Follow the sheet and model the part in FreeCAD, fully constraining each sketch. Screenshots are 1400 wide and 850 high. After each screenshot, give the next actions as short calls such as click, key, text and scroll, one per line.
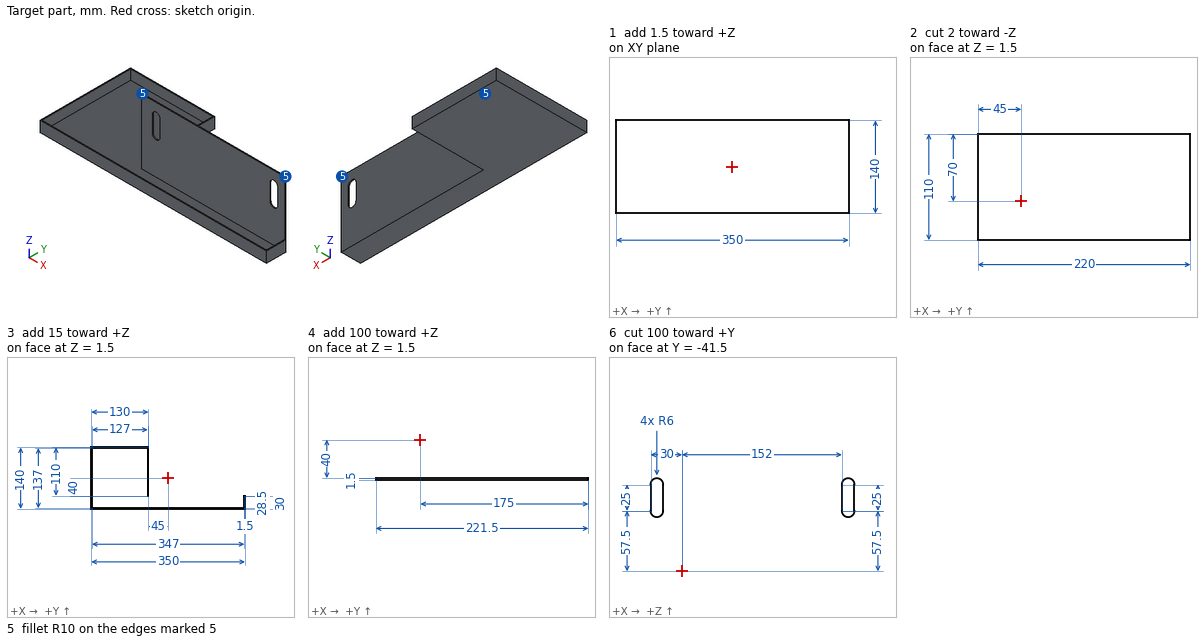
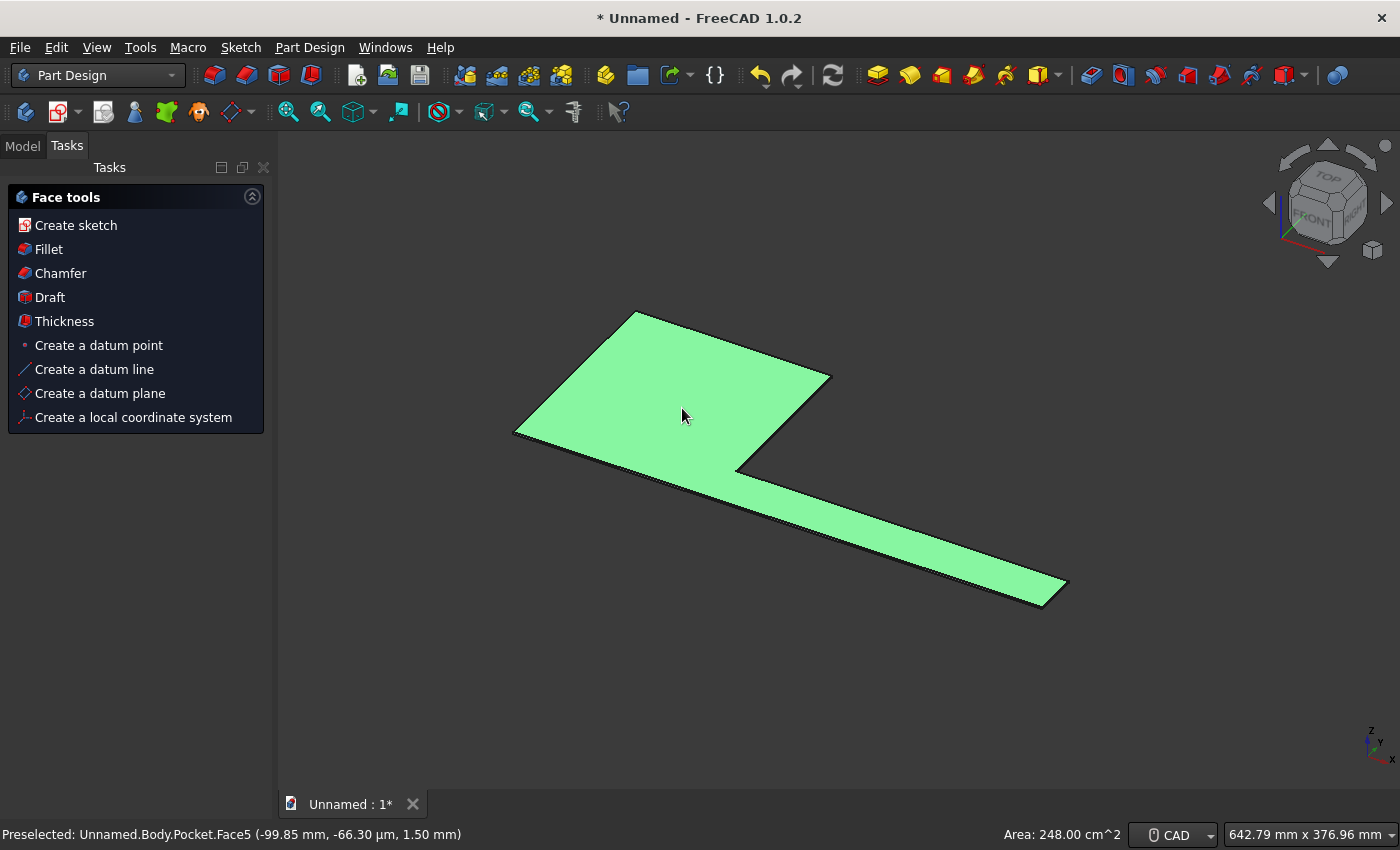
click(58, 112)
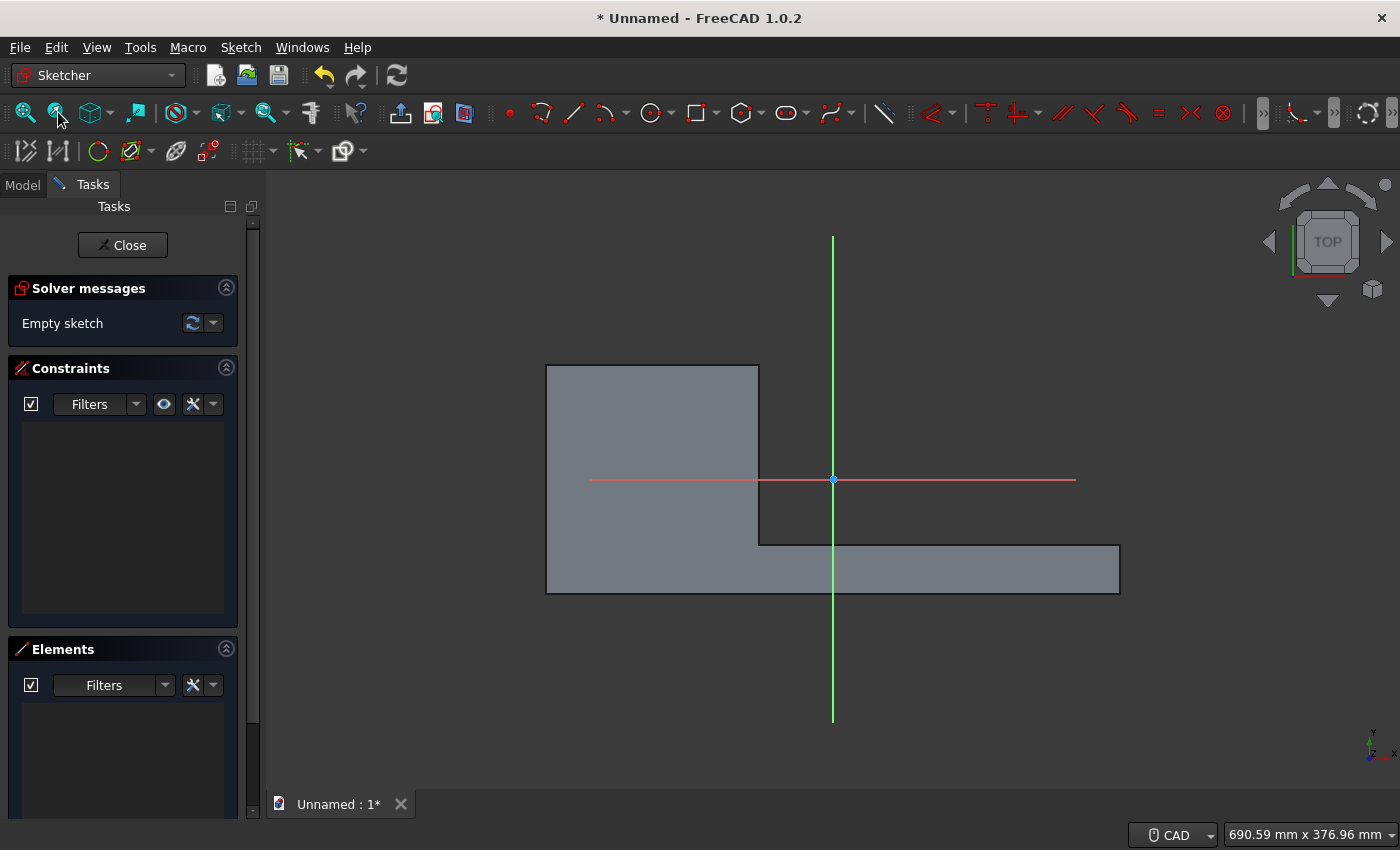
click(542, 114)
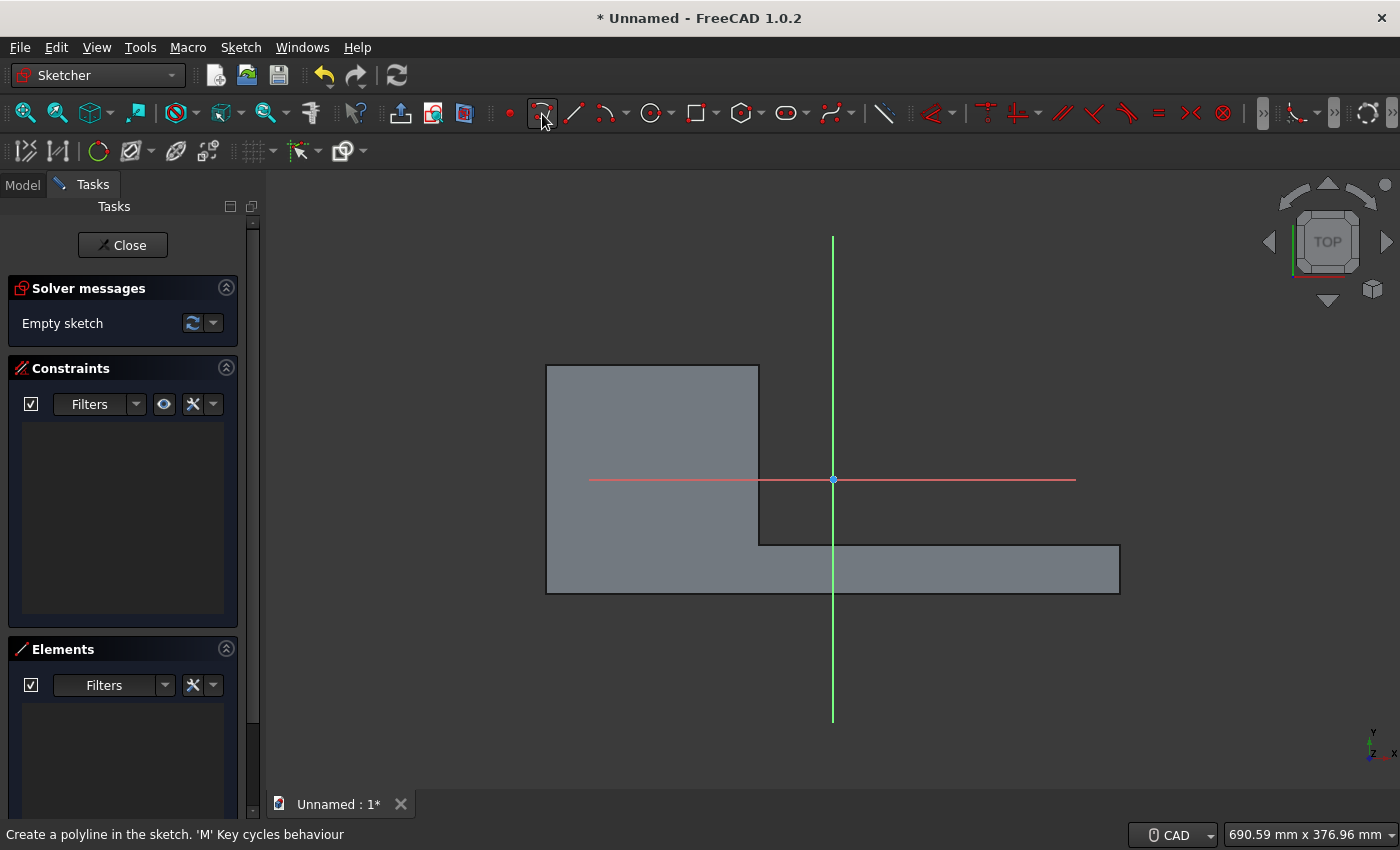
click(759, 545)
click(759, 365)
click(546, 365)
click(546, 594)
click(1120, 594)
click(1120, 545)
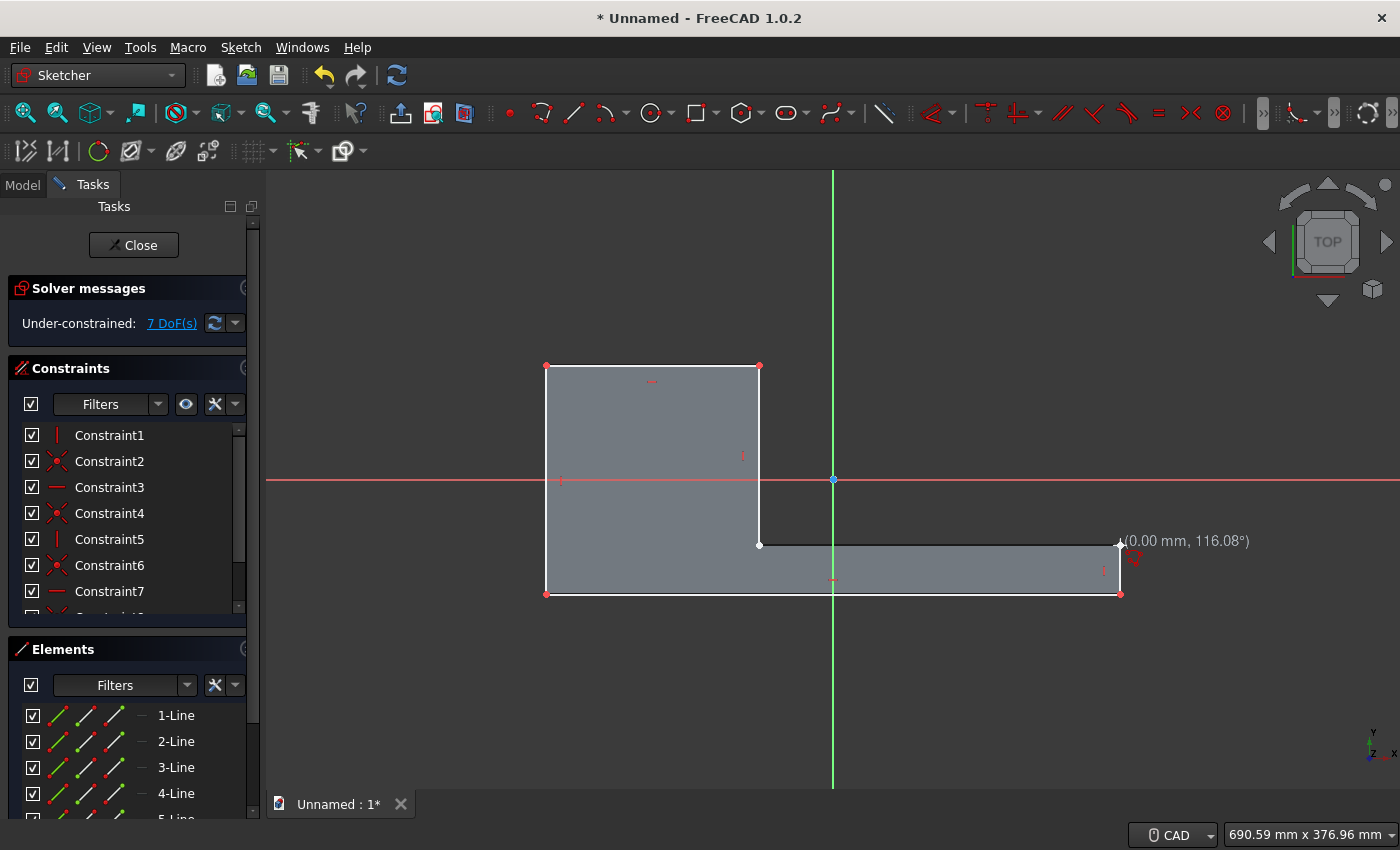
scroll(1118, 545, up, 10)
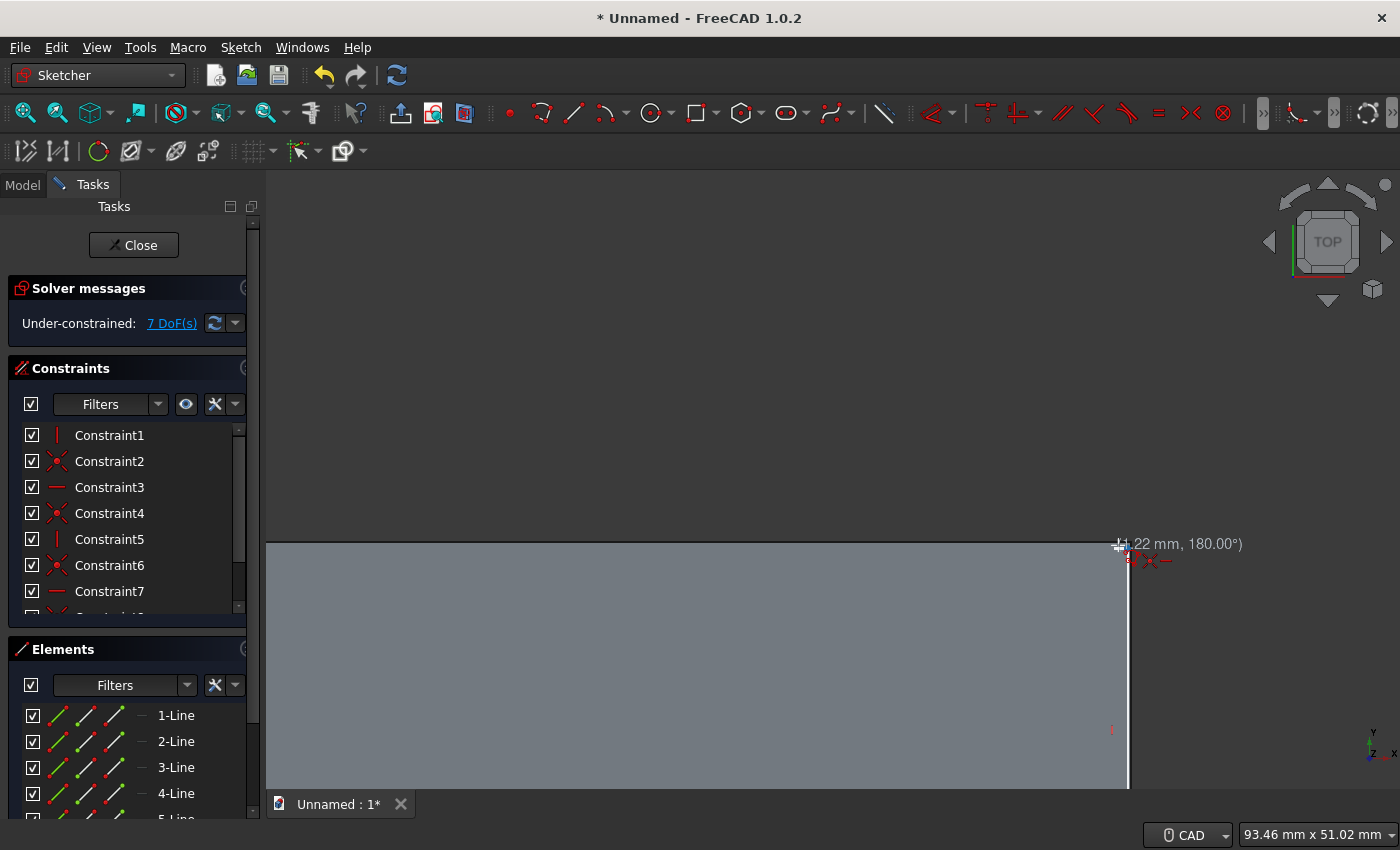
click(1112, 541)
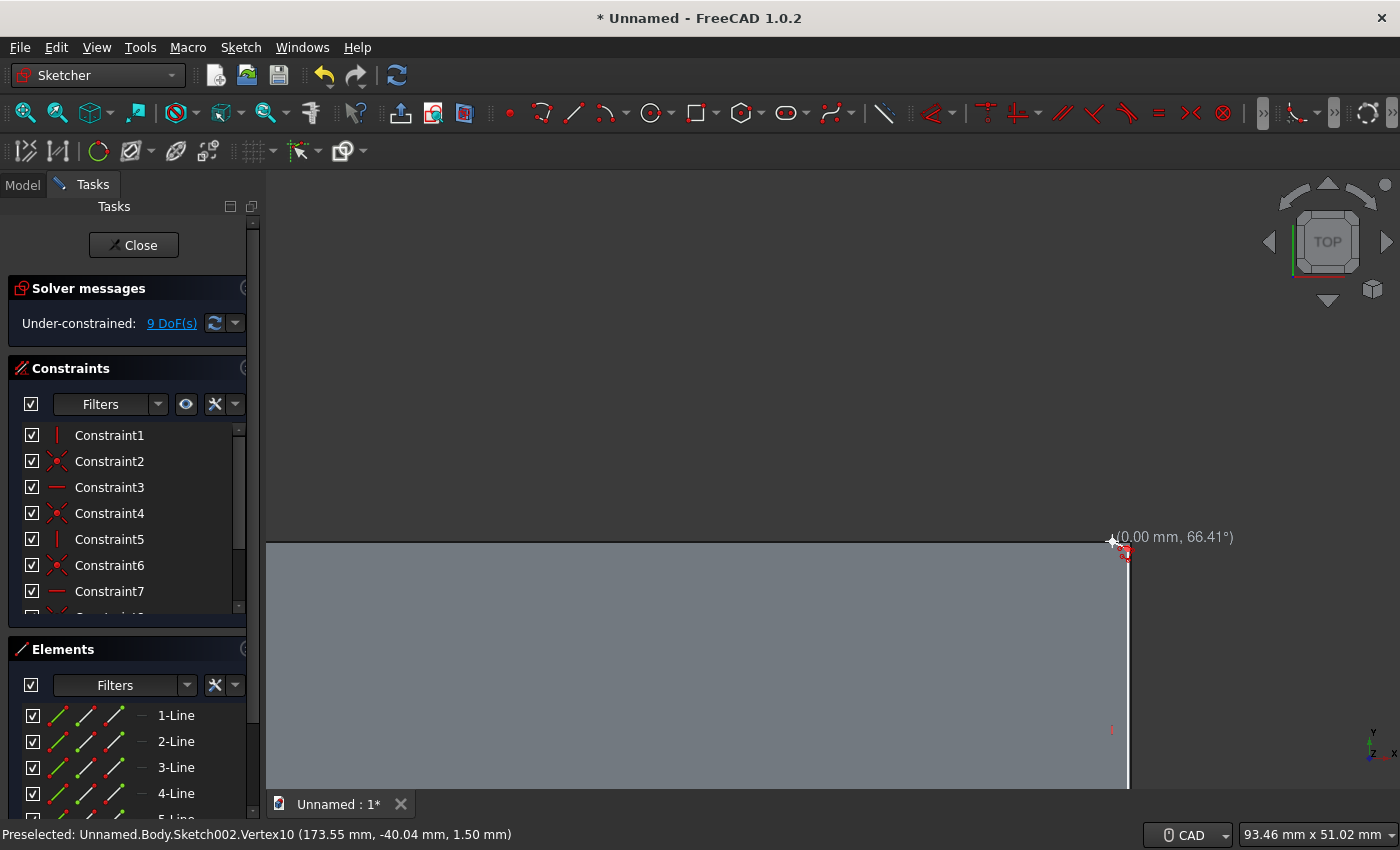
scroll(1112, 563, down, 9)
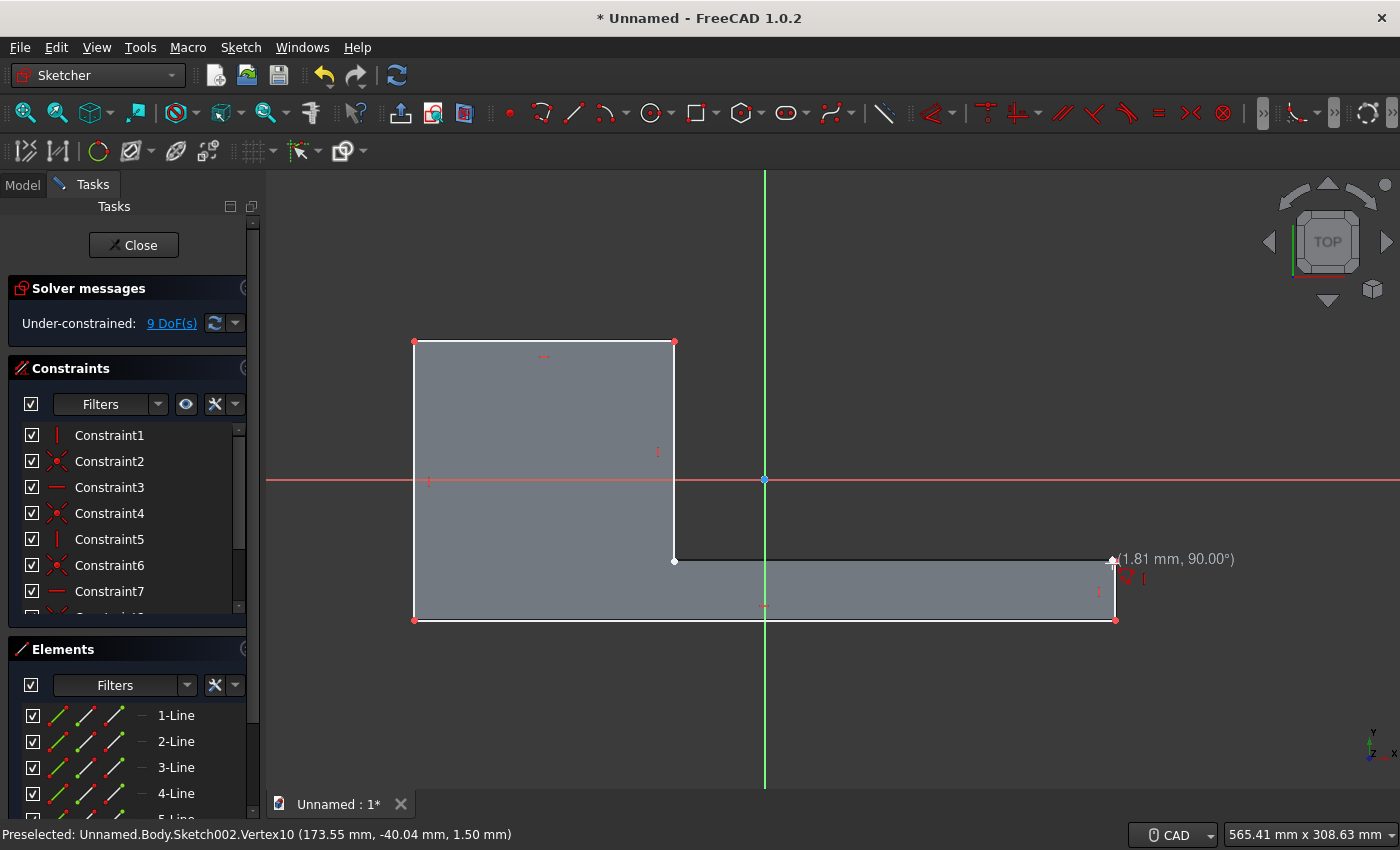
scroll(1113, 617, up, 9)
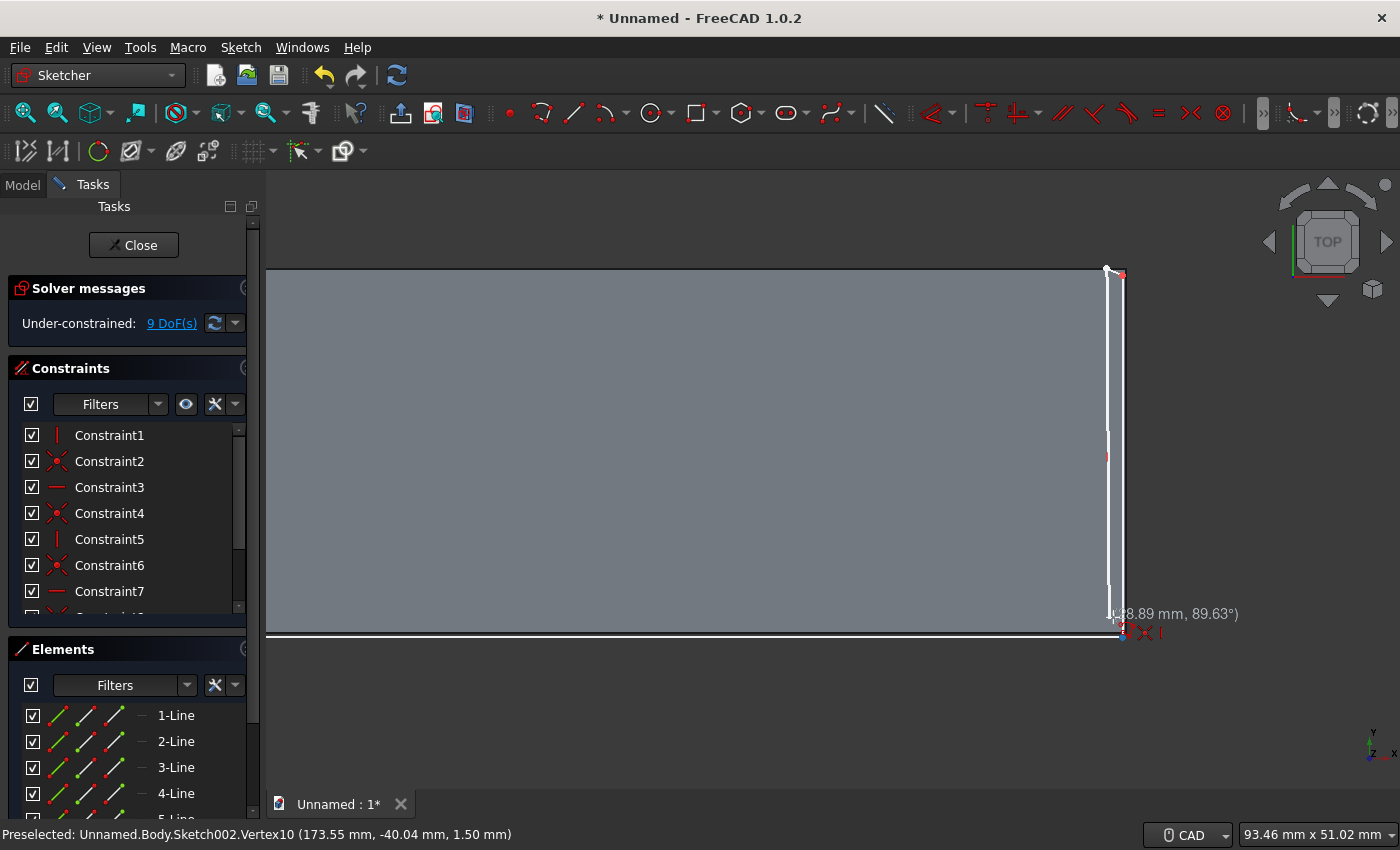
click(1107, 615)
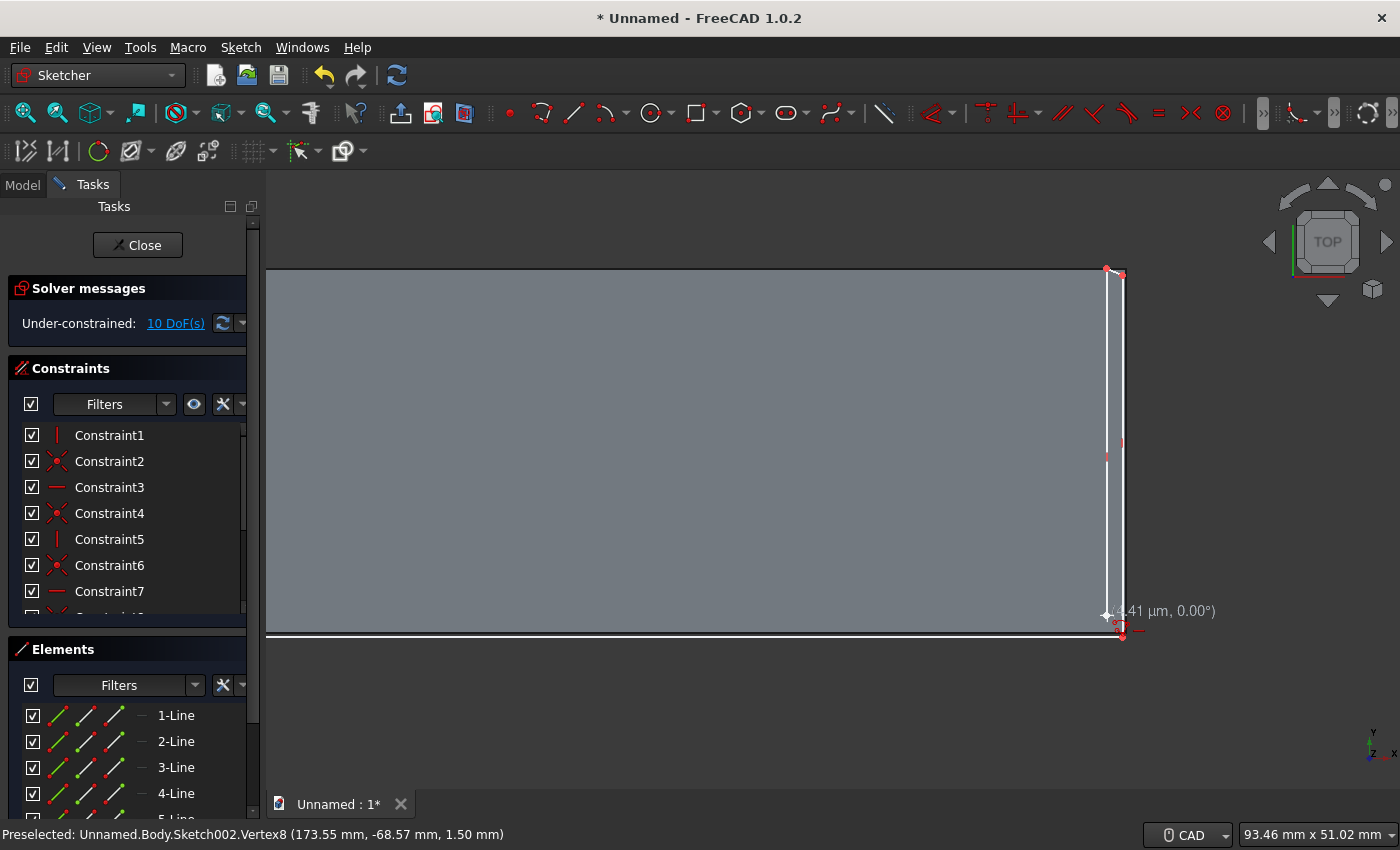
scroll(1113, 617, down, 9)